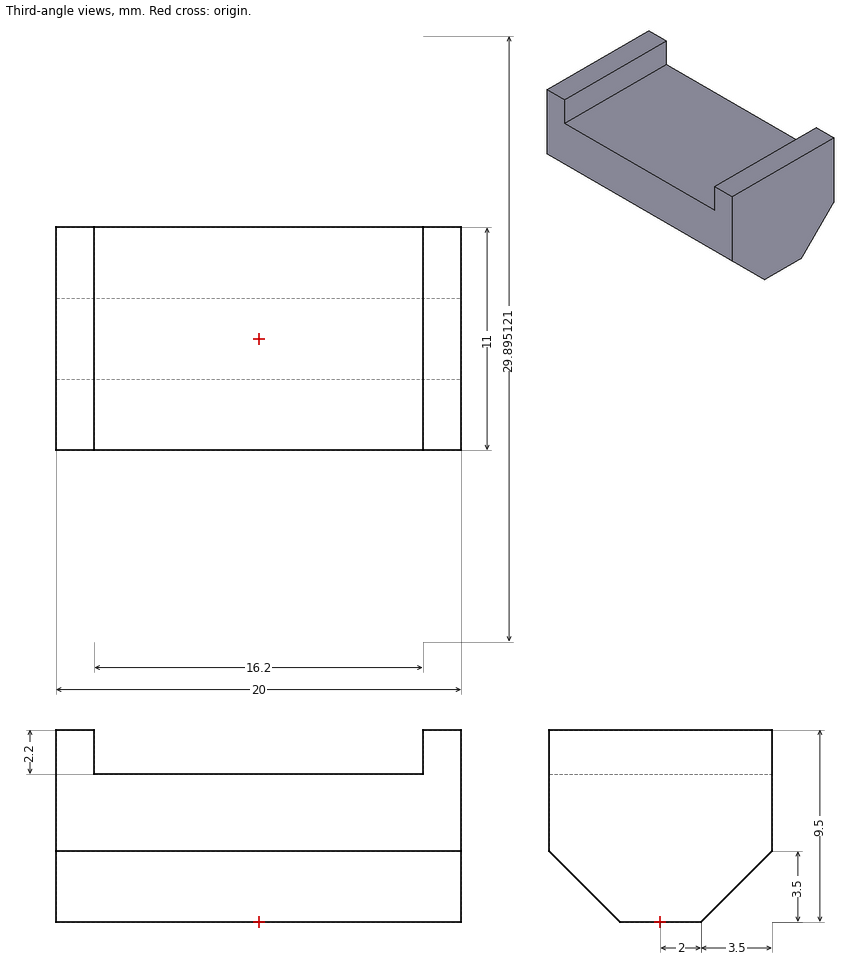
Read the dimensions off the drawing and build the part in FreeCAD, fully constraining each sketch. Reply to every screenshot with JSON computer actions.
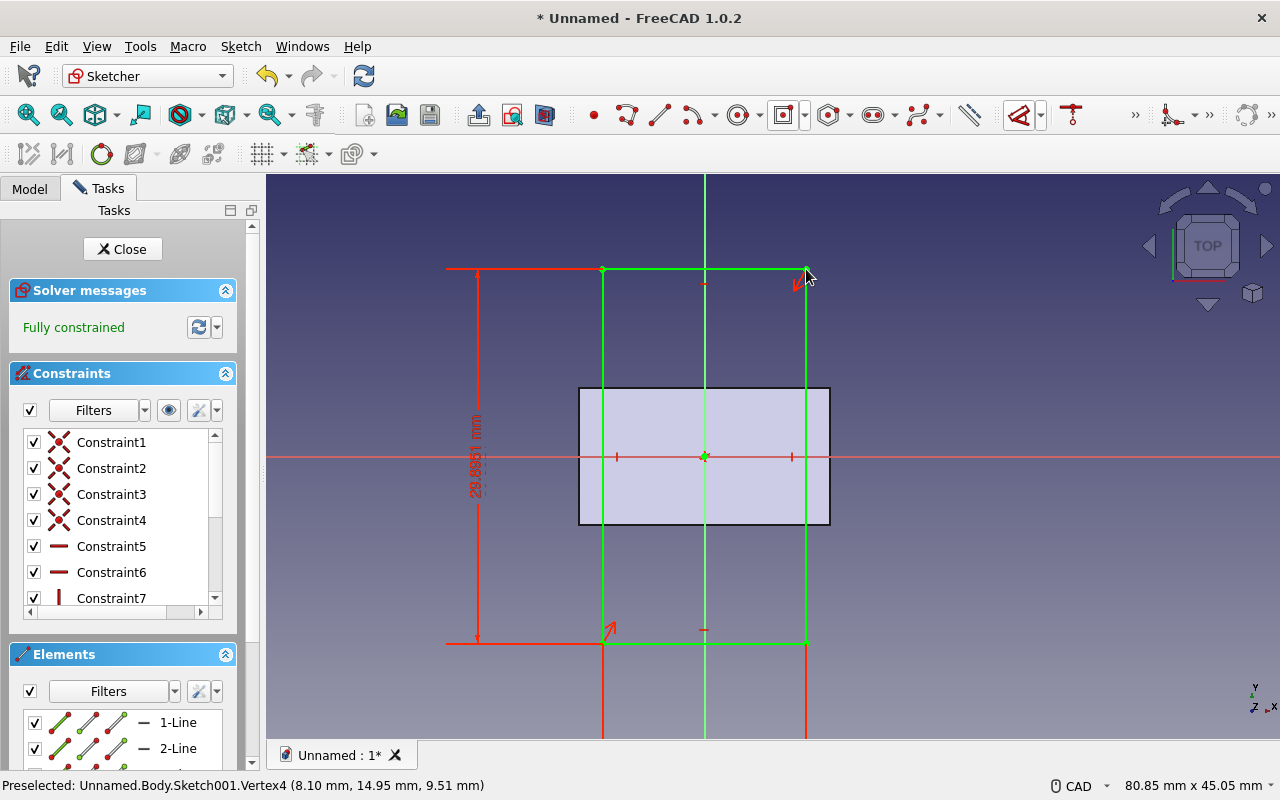
{"action": "left_click", "coordinate": [123, 249]}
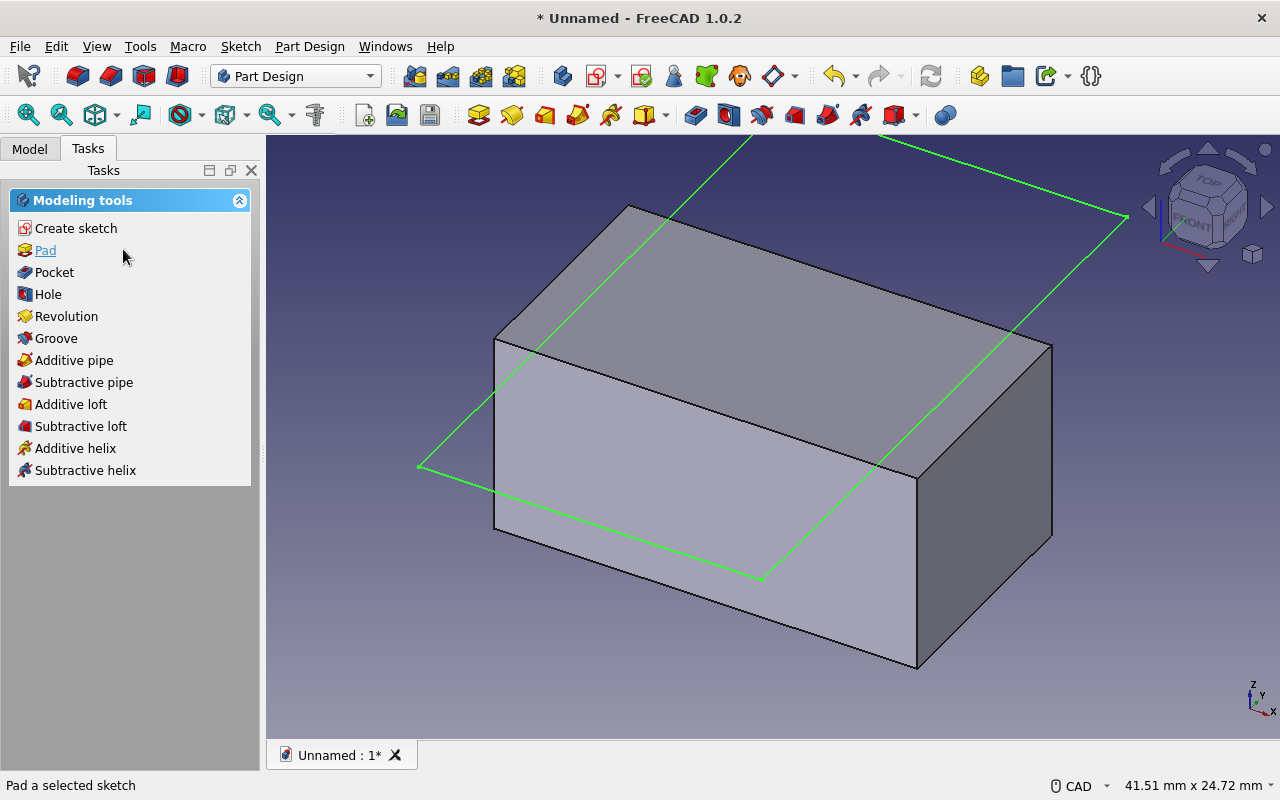
{"action": "left_click", "coordinate": [696, 116]}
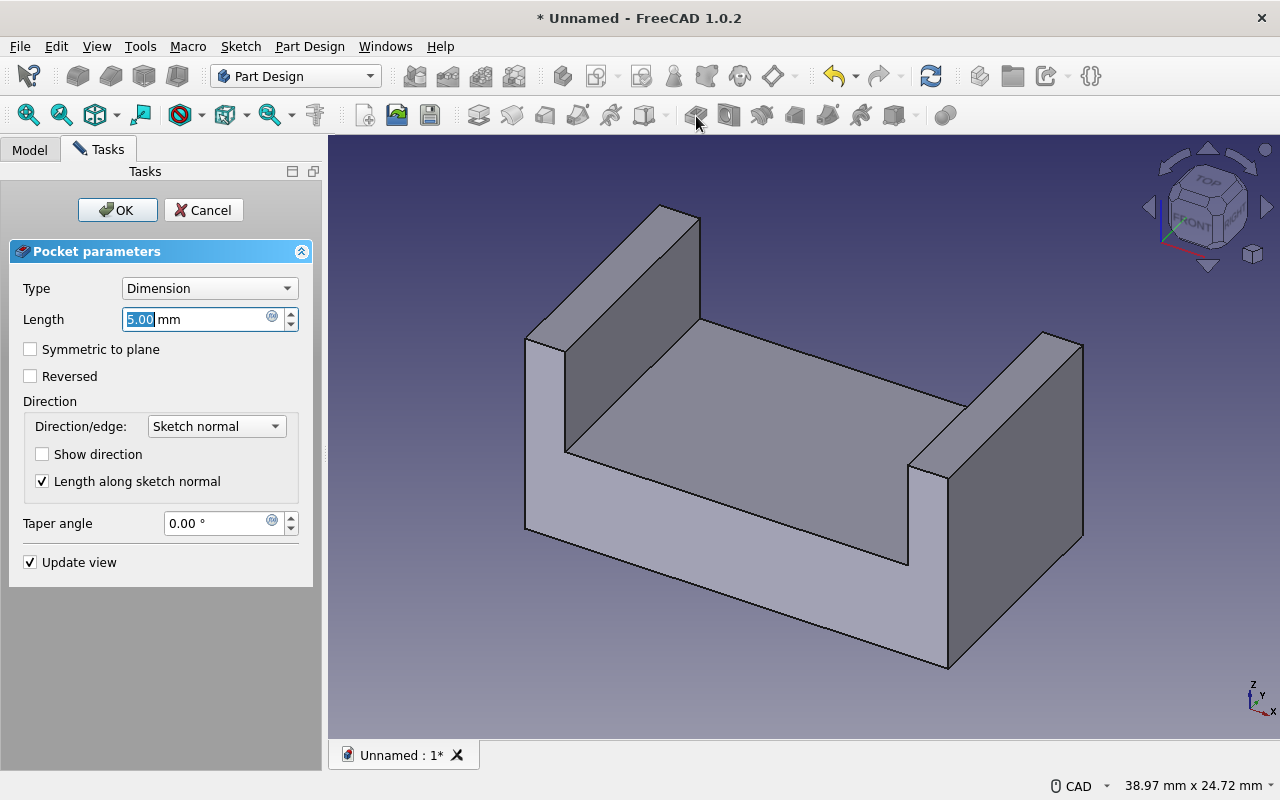
{"action": "type", "text": "2.2"}
{"action": "key", "text": "Tab"}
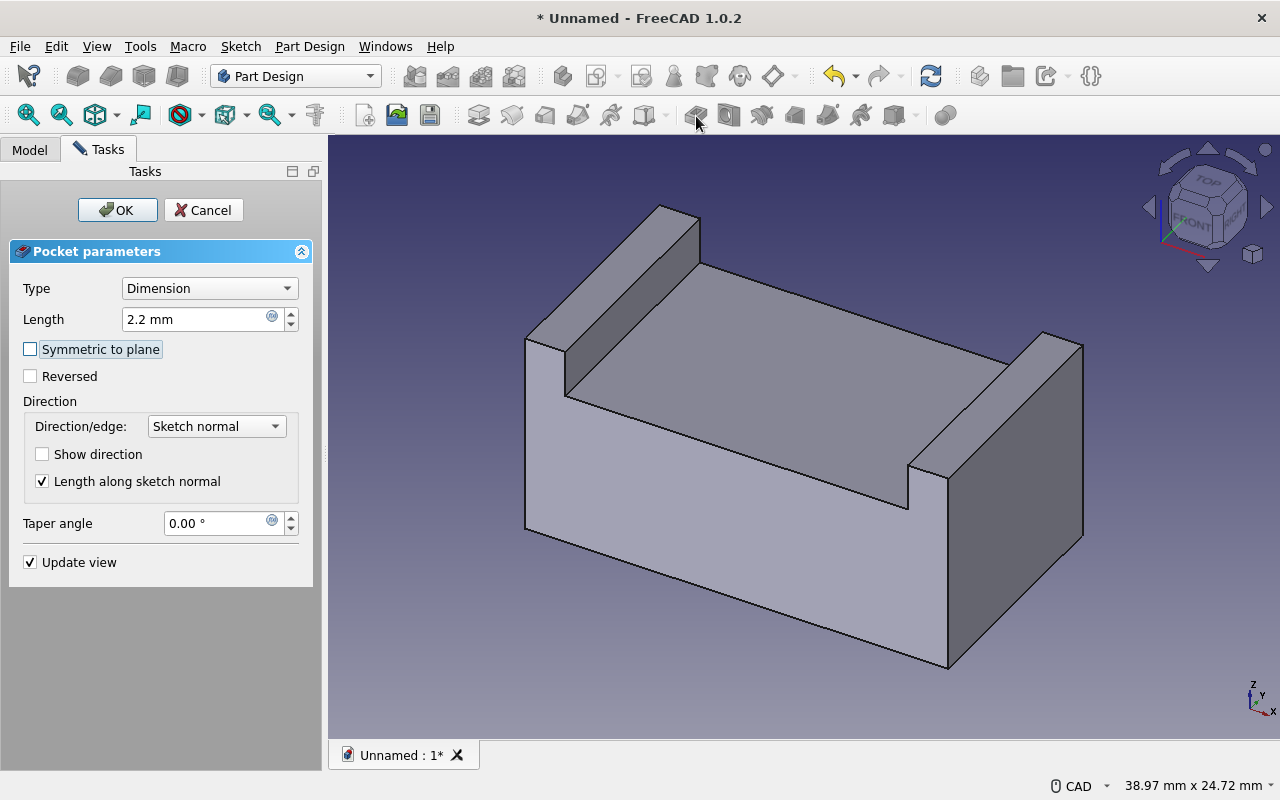
{"action": "left_click", "coordinate": [118, 210]}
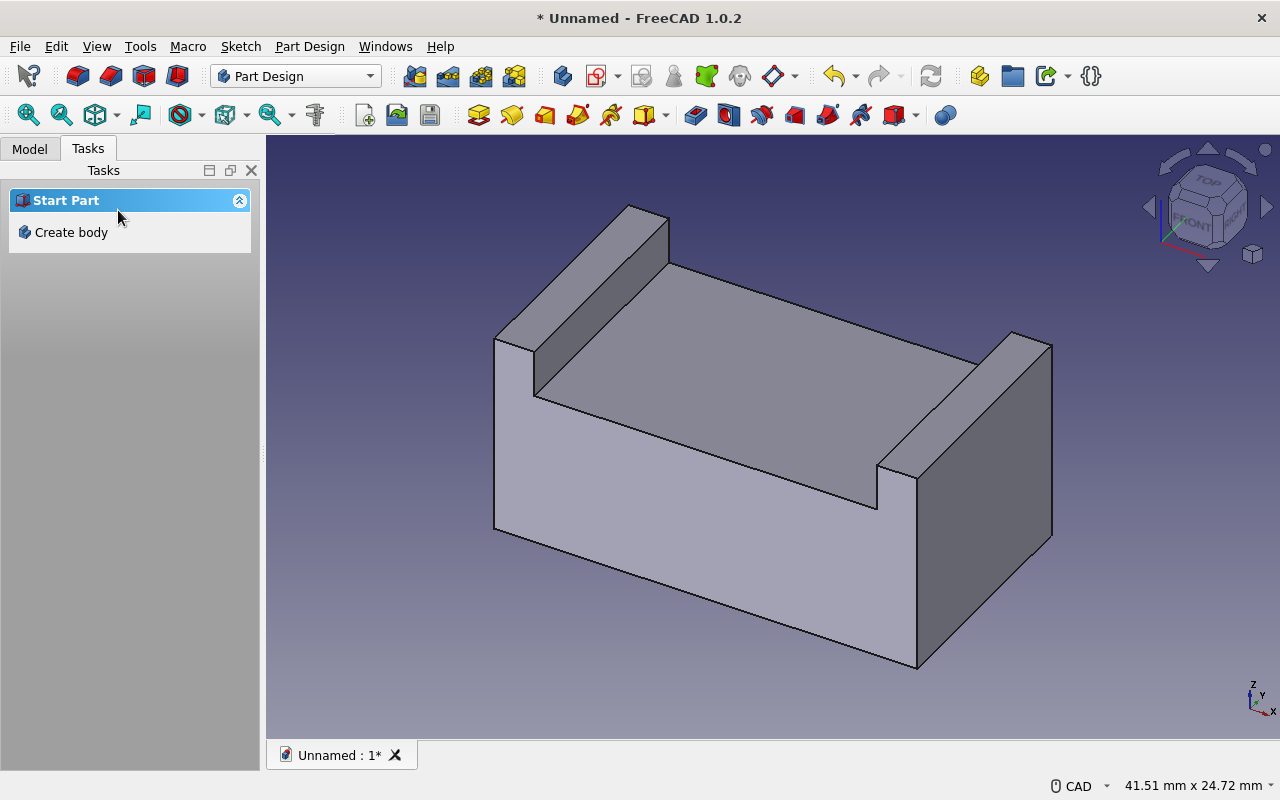
{"action": "key", "text": "6"}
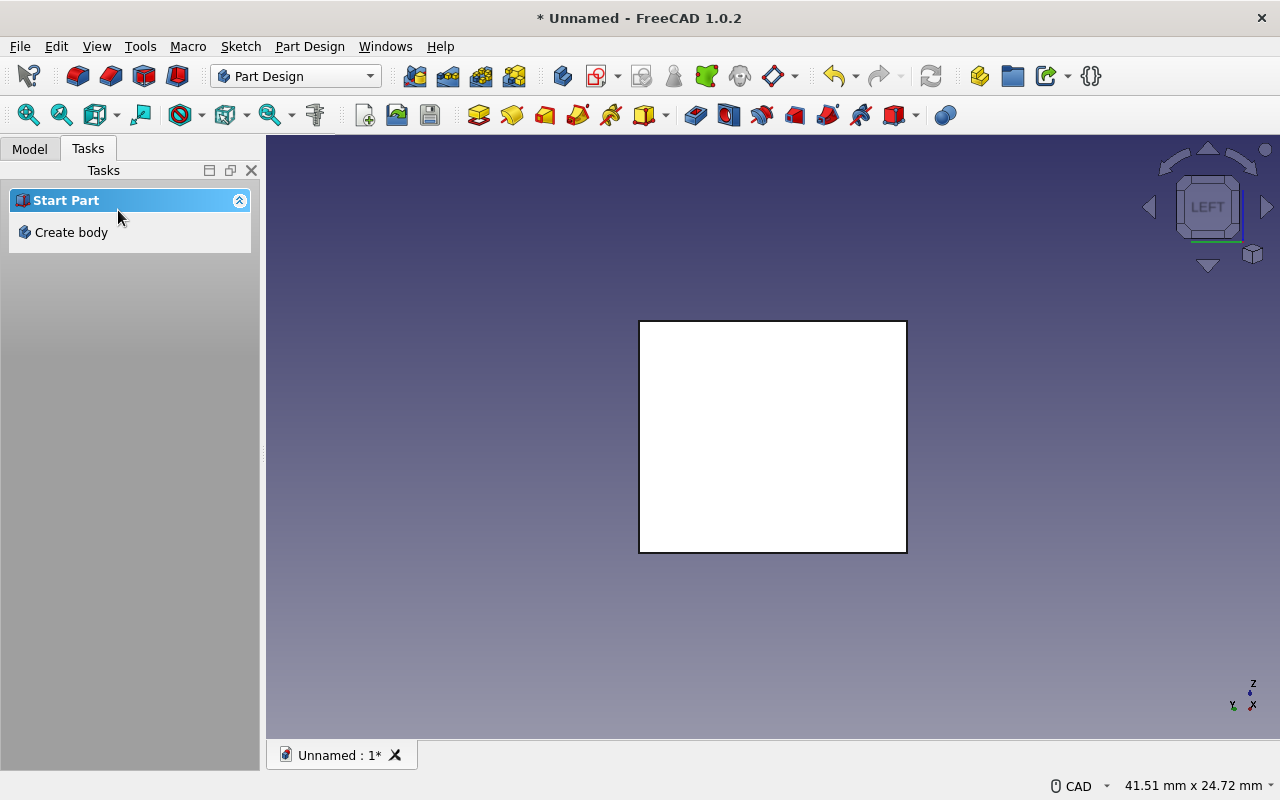
{"action": "left_click", "coordinate": [29, 116]}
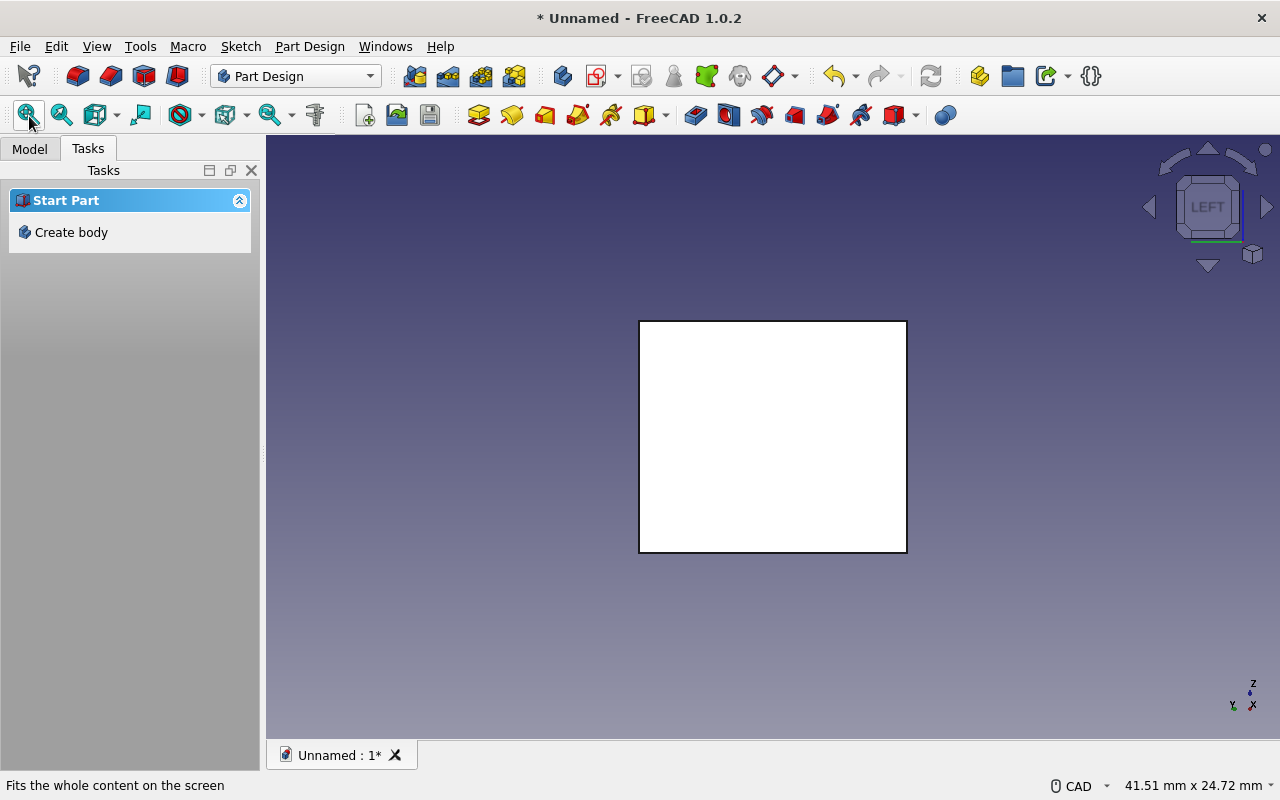
{"action": "left_click", "coordinate": [773, 436]}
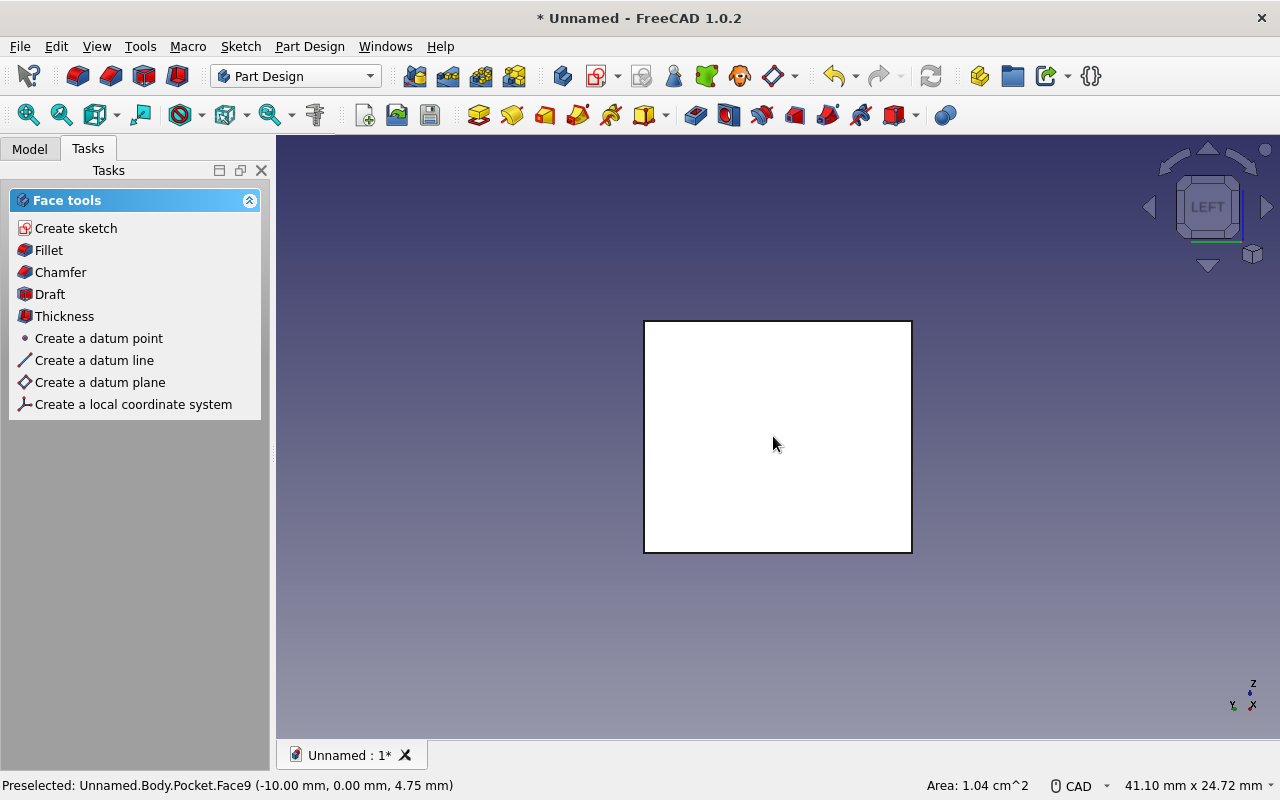
{"action": "left_click", "coordinate": [596, 76]}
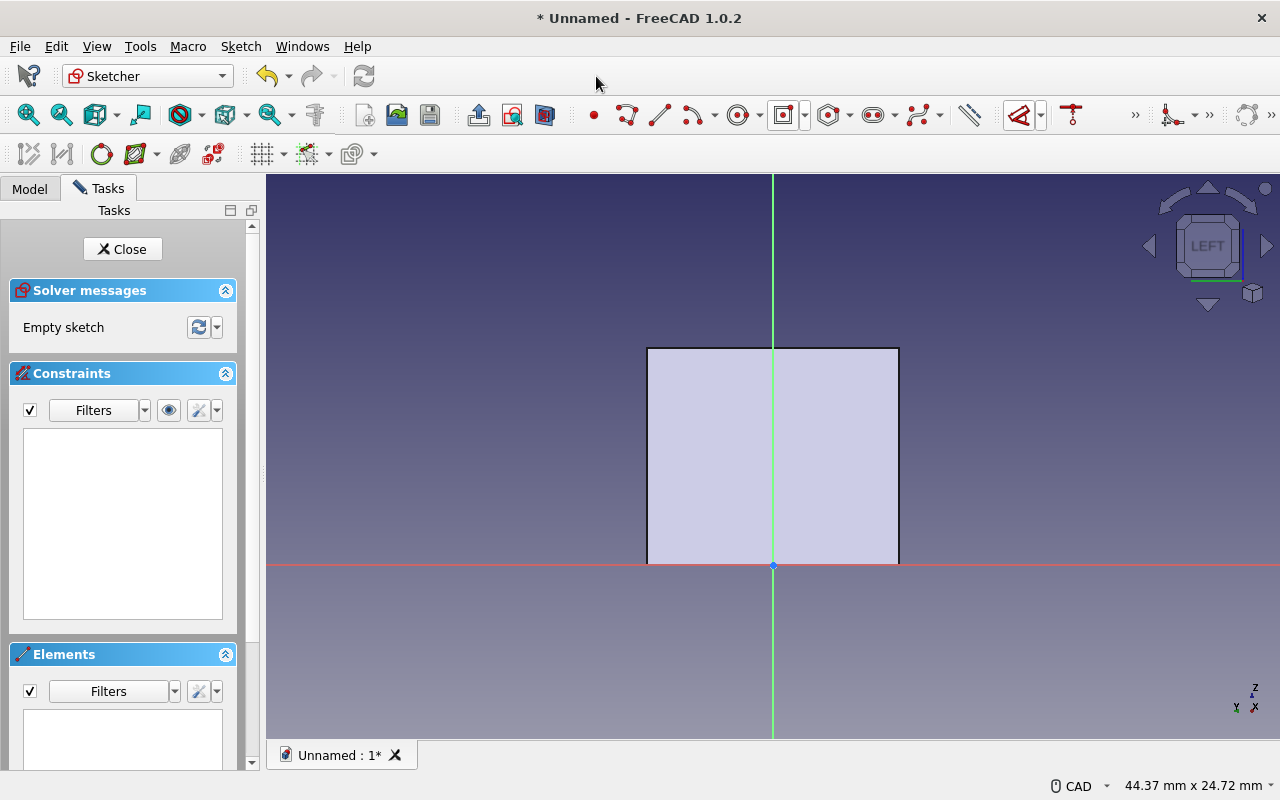
{"action": "scroll", "coordinate": [712, 542], "scroll_direction": "up", "scroll_amount": 8}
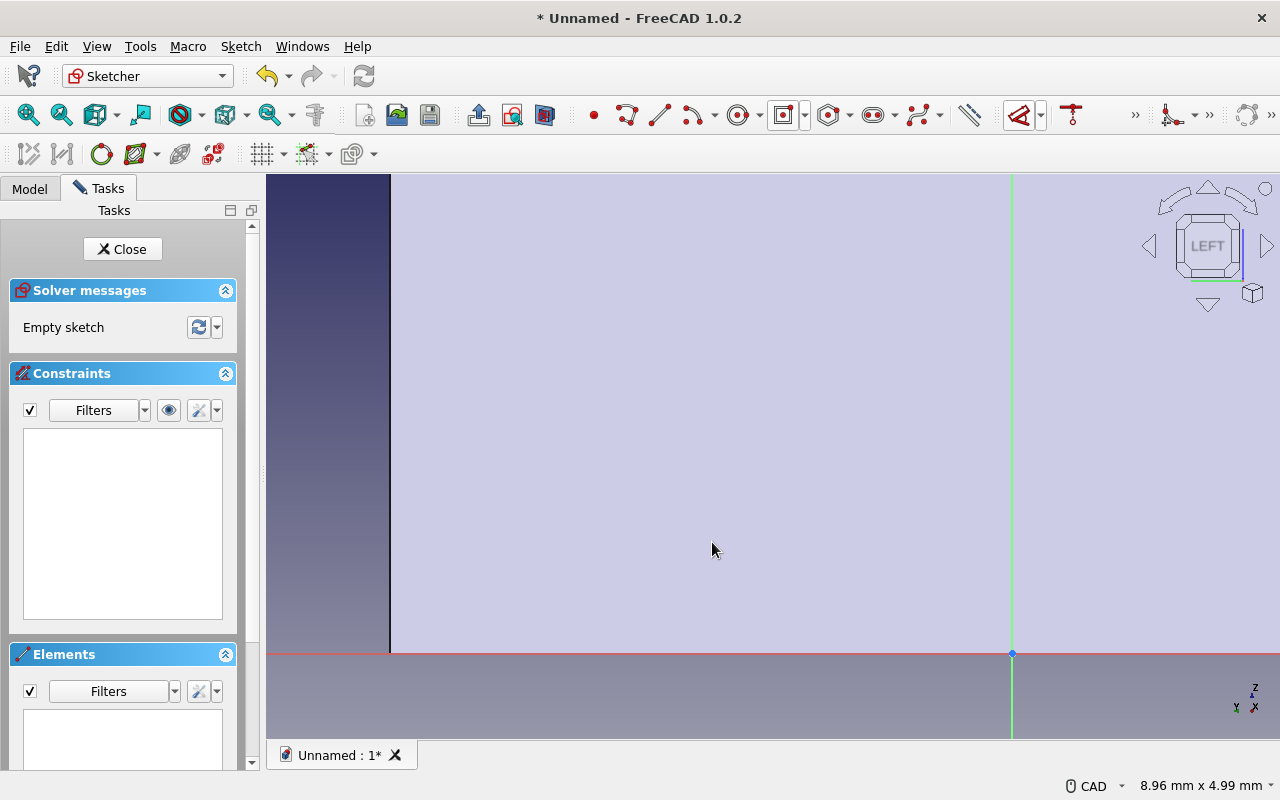
{"action": "left_click", "coordinate": [627, 116]}